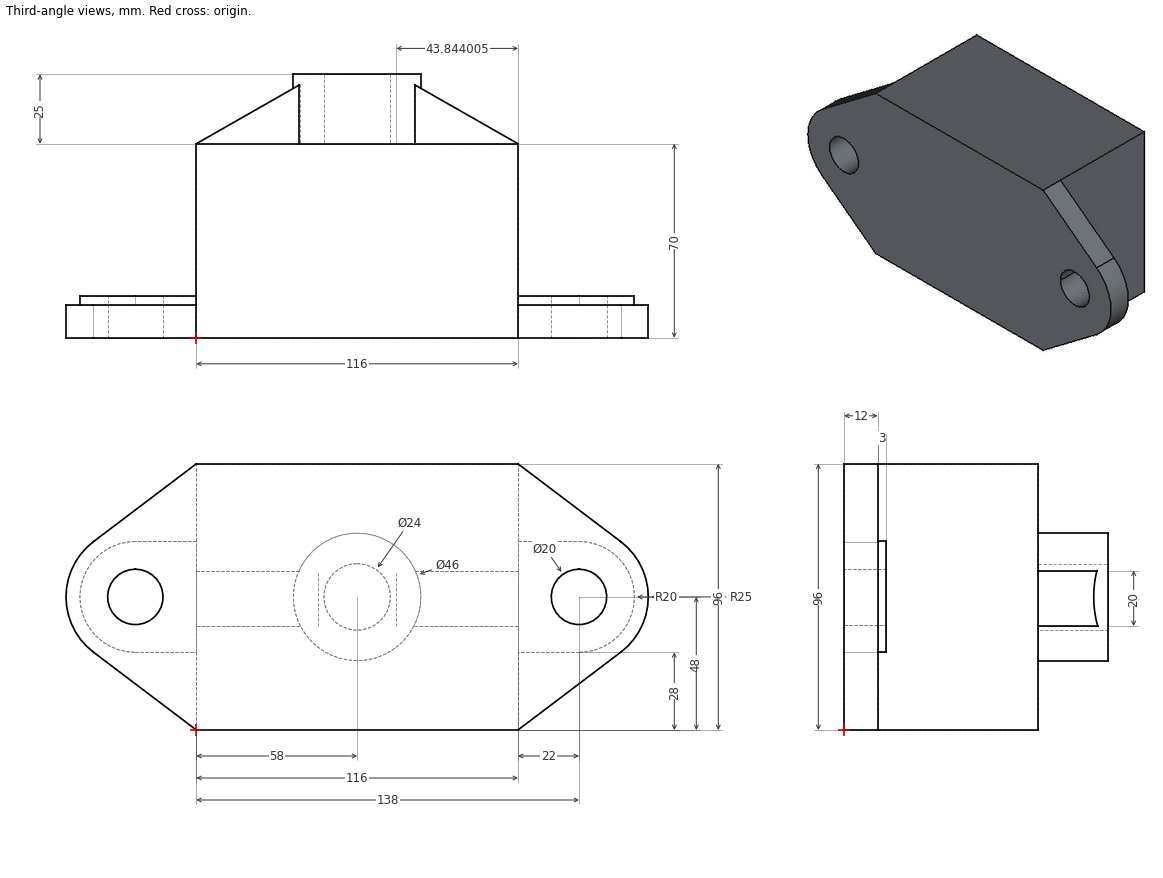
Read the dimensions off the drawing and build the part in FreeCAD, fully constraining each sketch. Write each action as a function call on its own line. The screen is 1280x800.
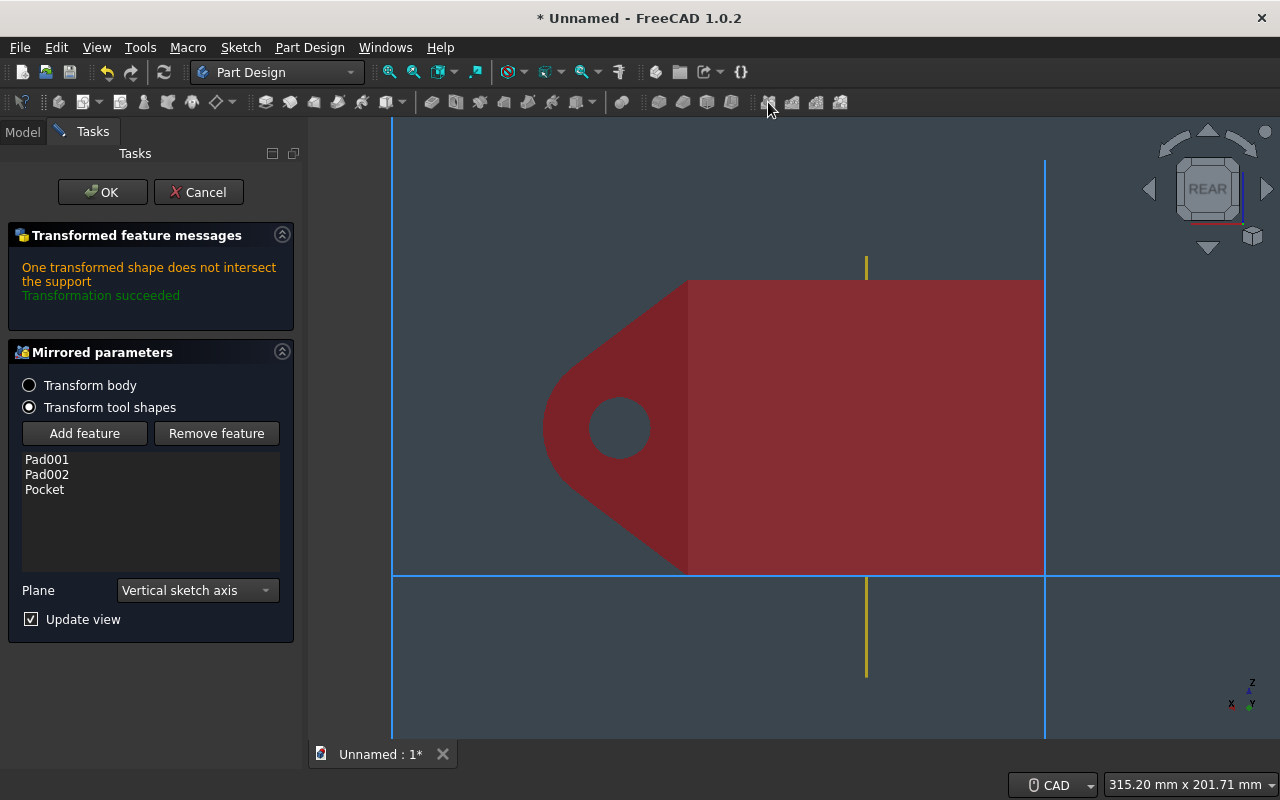
click(198, 590)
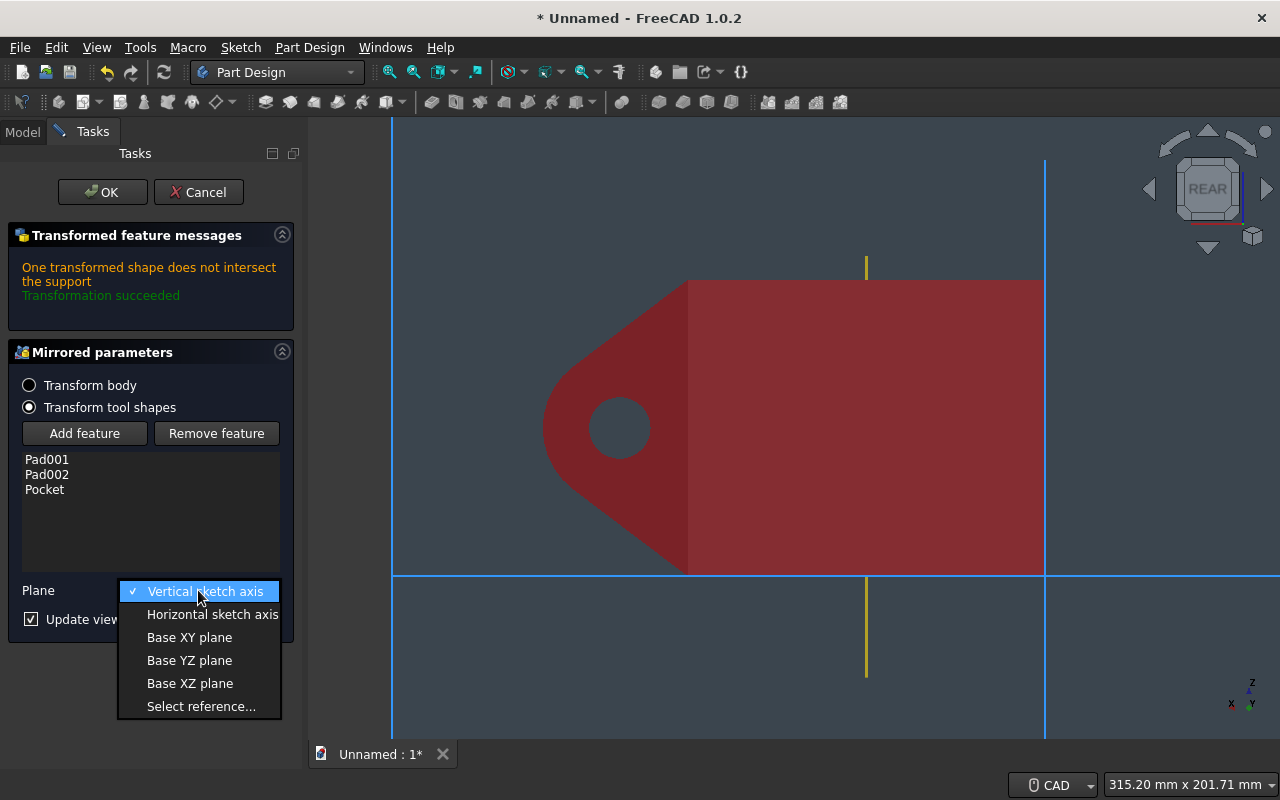
click(198, 706)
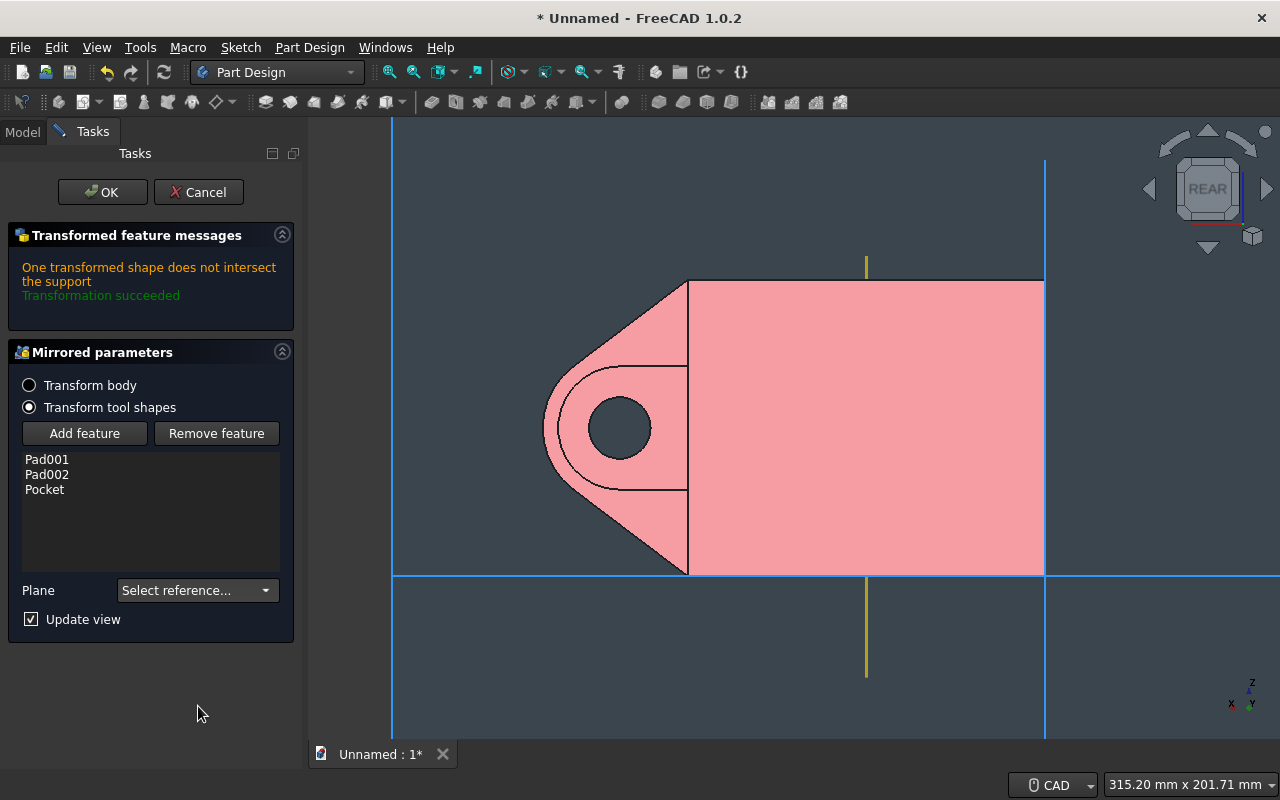
click(23, 131)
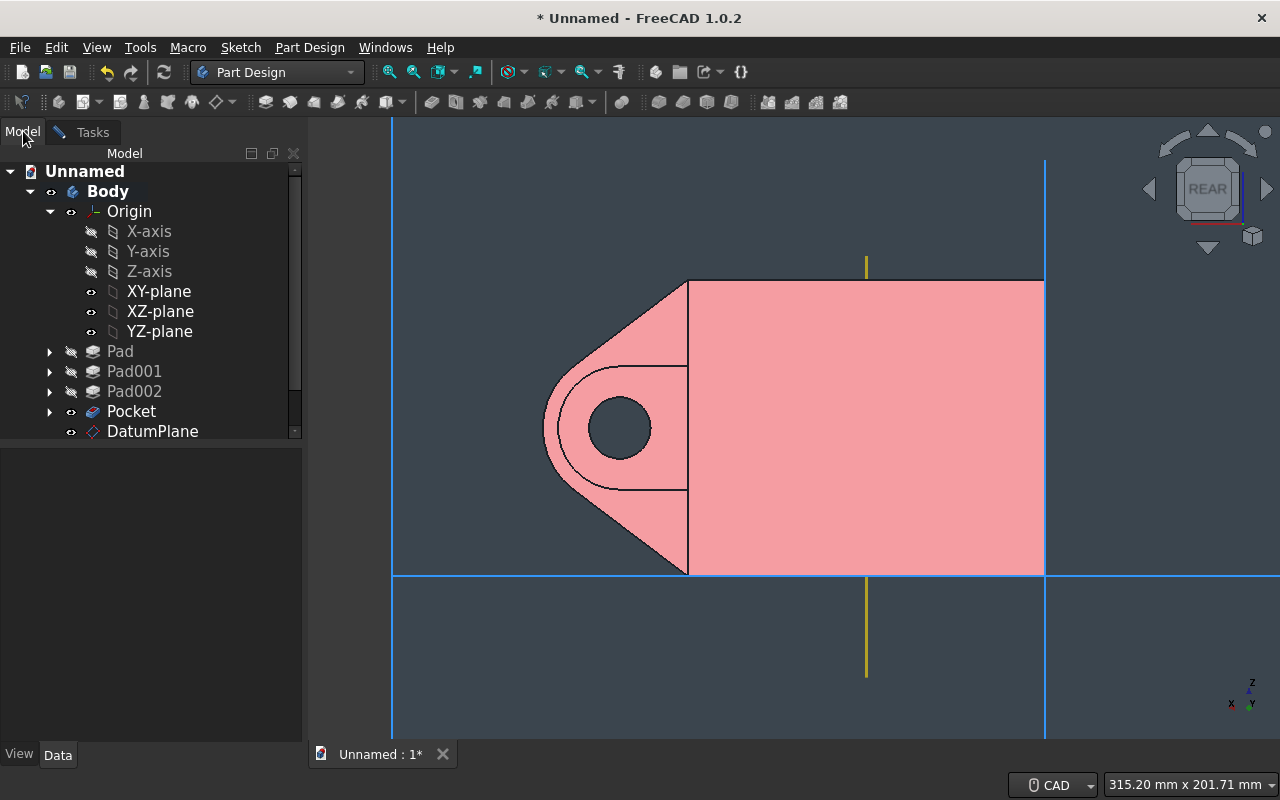
click(116, 432)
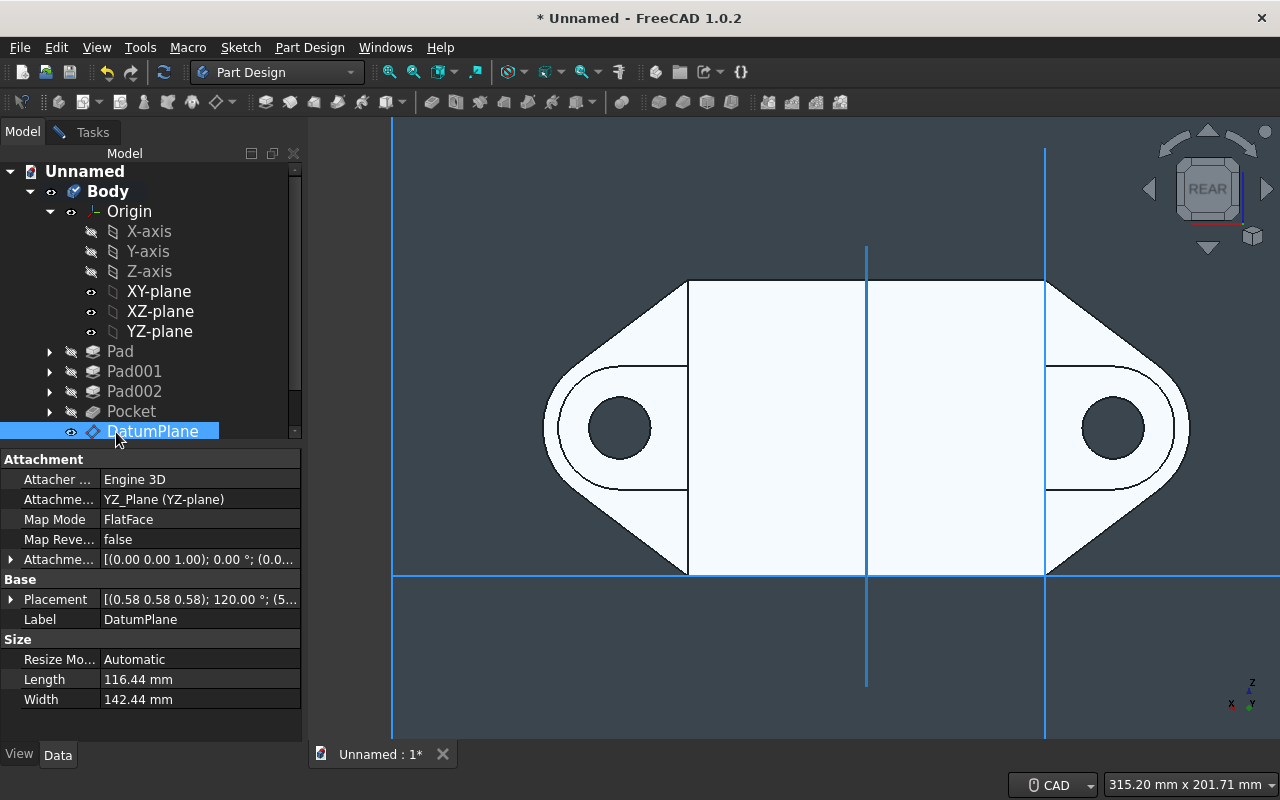
click(84, 131)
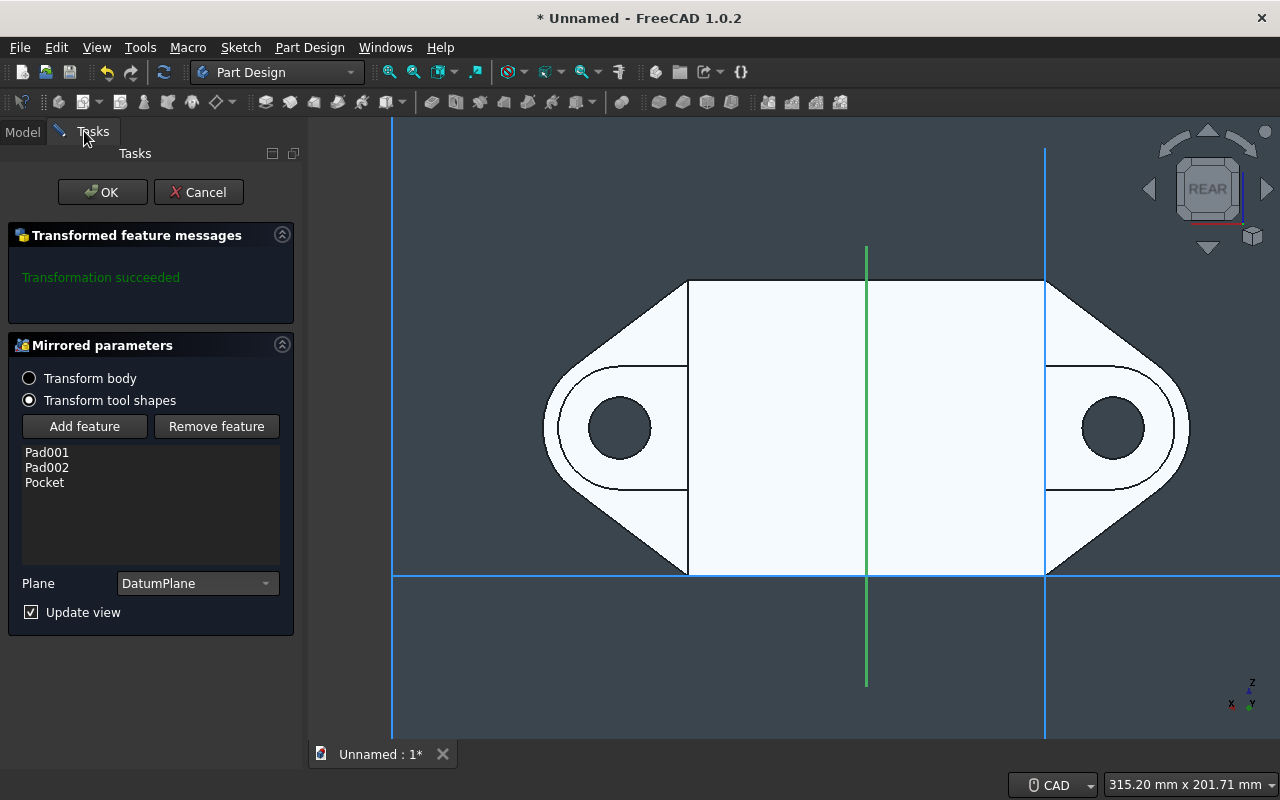
click(103, 192)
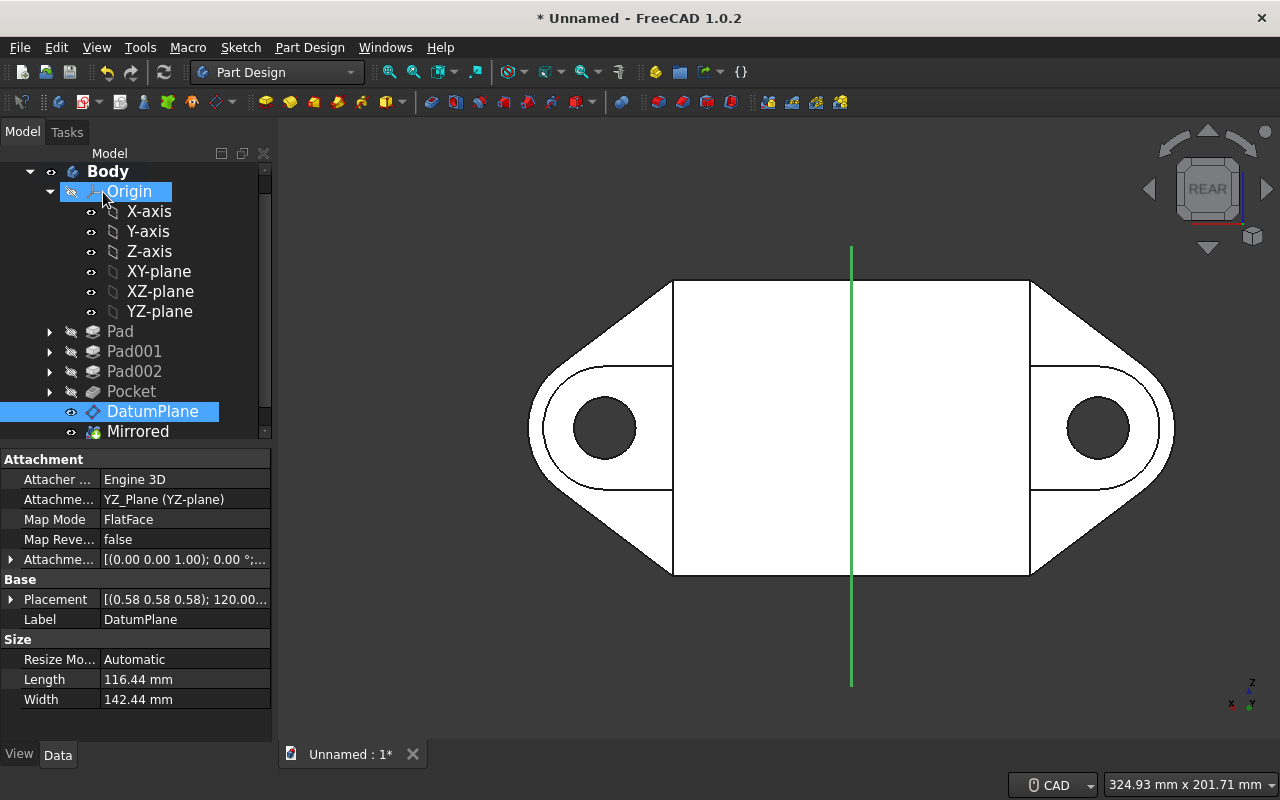
click(116, 412)
key(space)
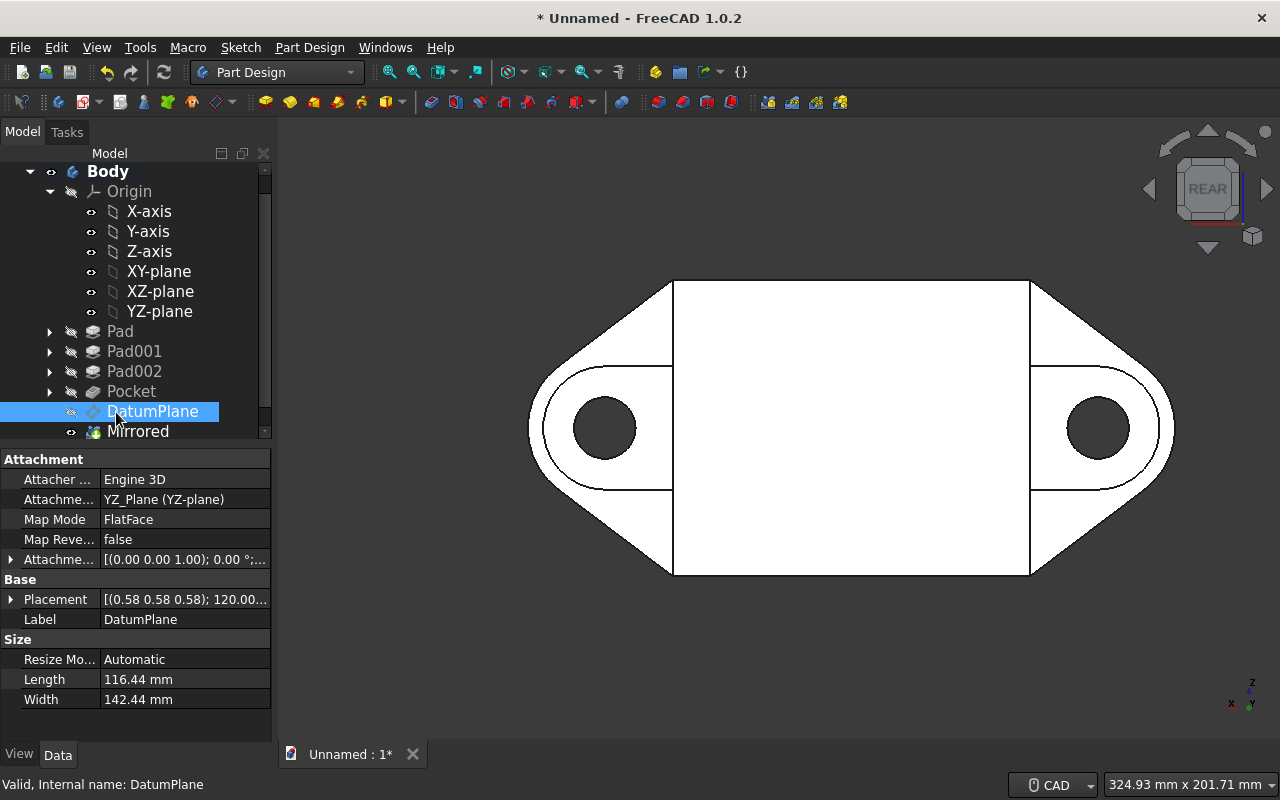
click(851, 427)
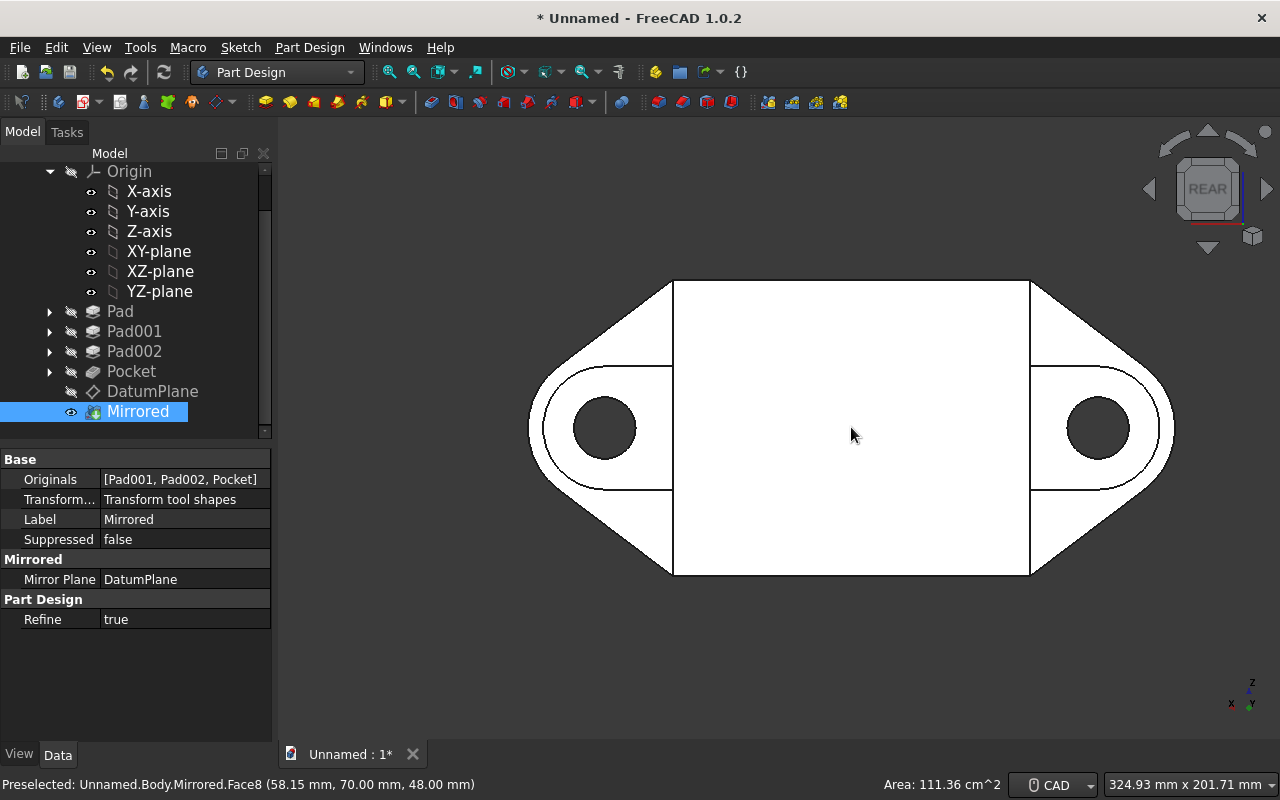
click(84, 102)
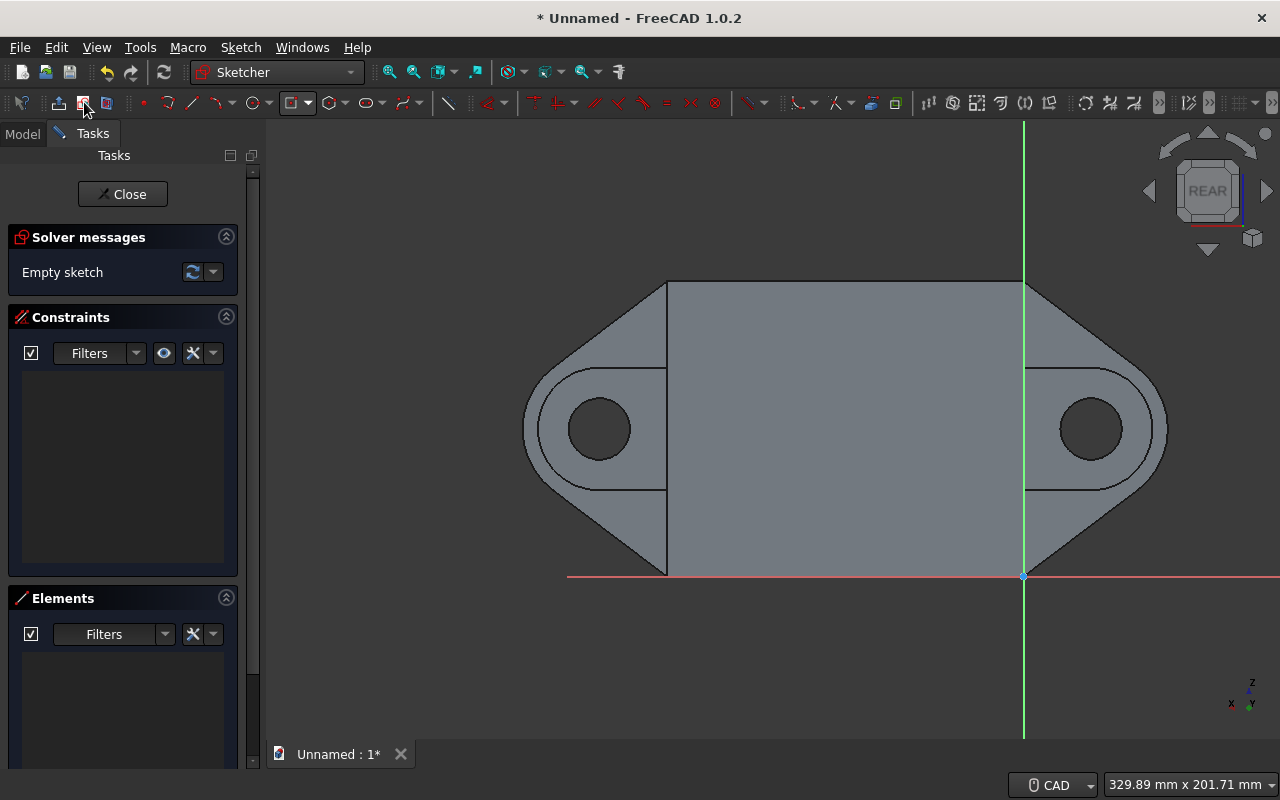
scroll(1115, 514, up, 3)